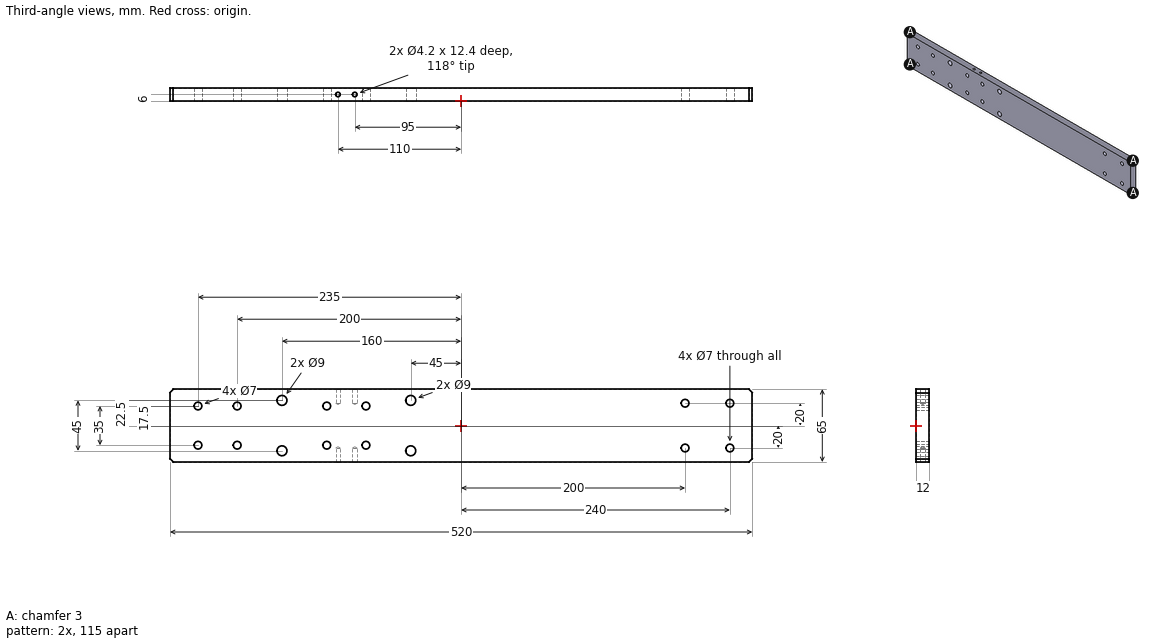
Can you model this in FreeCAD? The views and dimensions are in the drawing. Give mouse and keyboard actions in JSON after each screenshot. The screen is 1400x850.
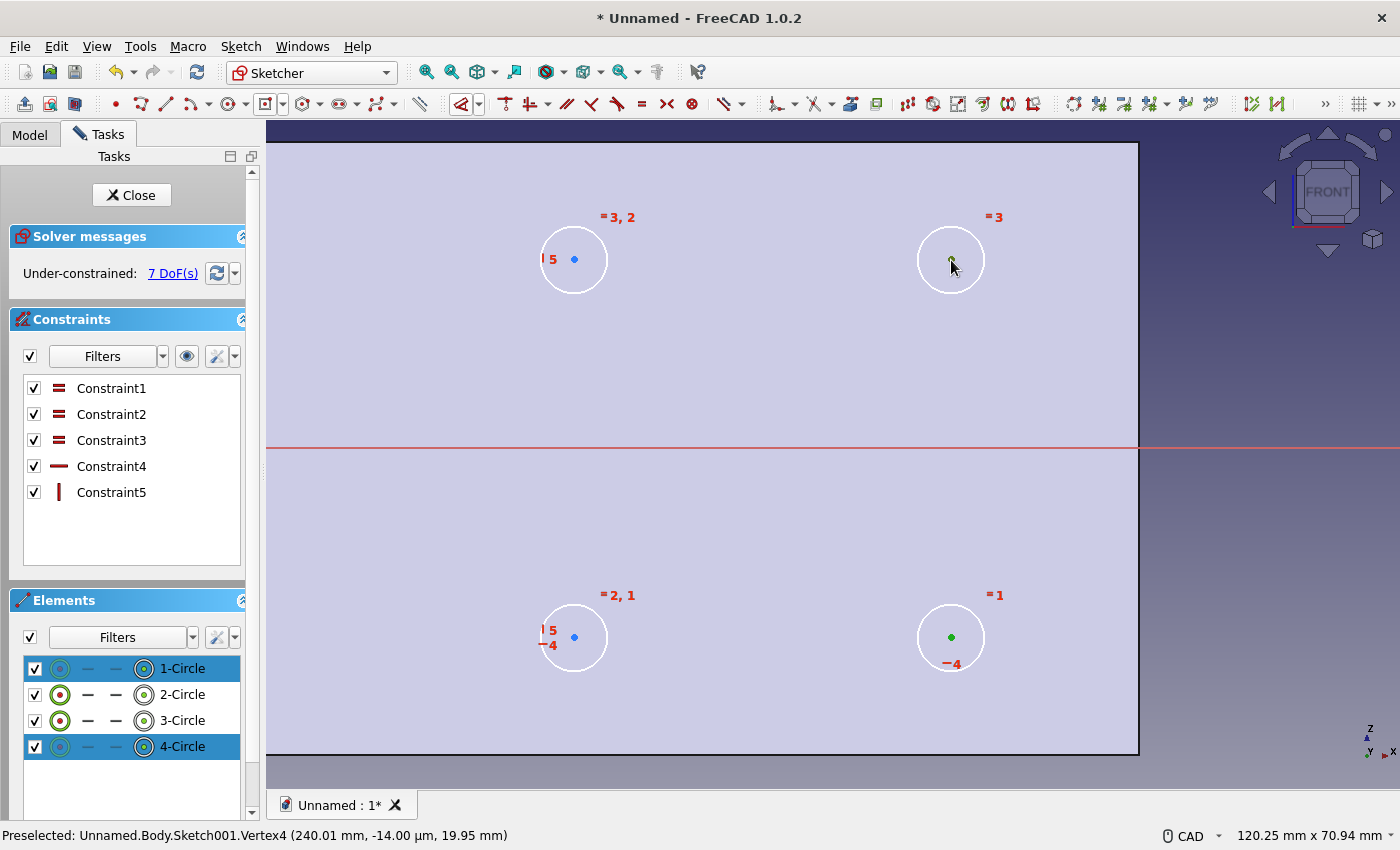
{"action": "left_click", "coordinate": [548, 104]}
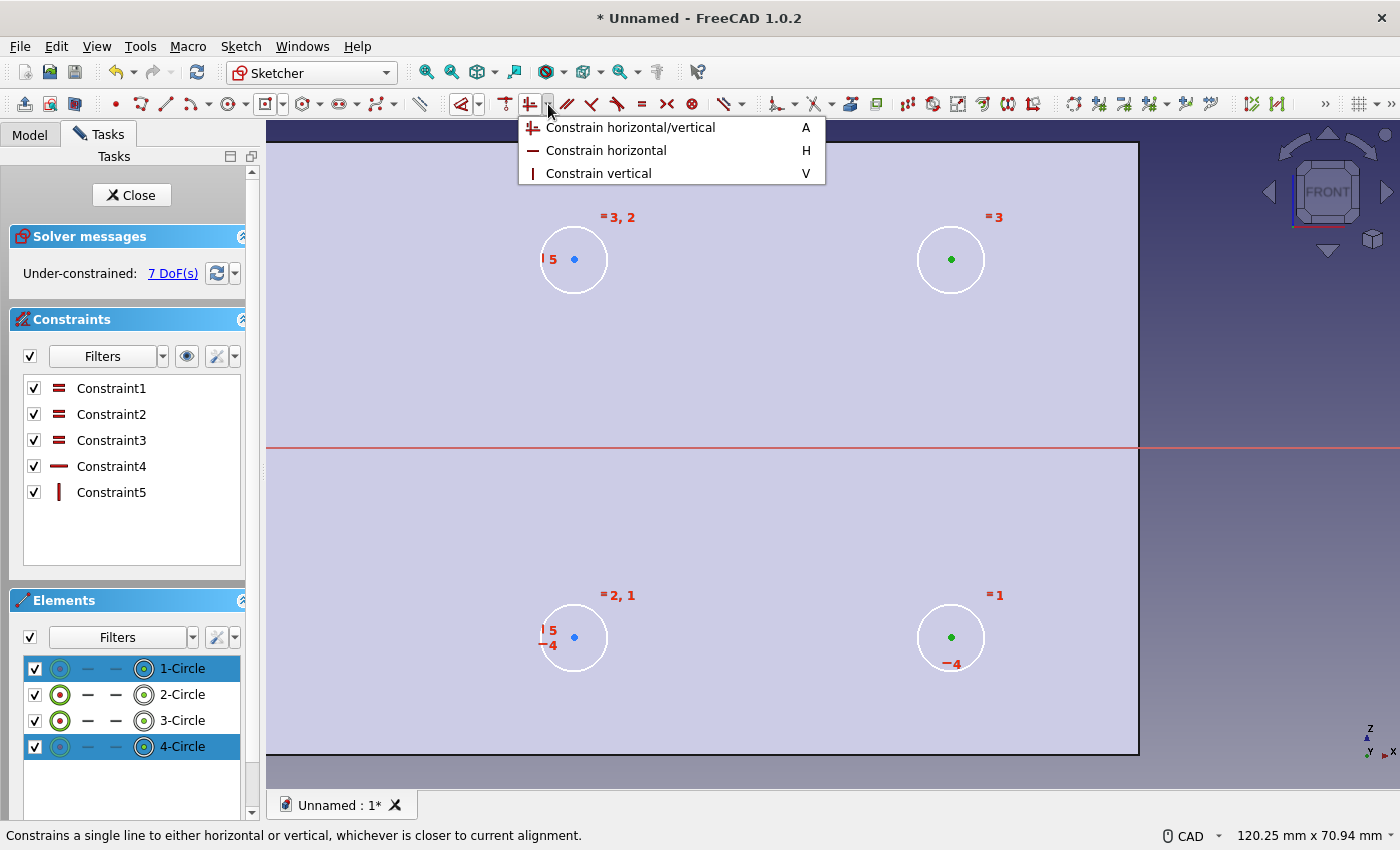
{"action": "left_click", "coordinate": [672, 174]}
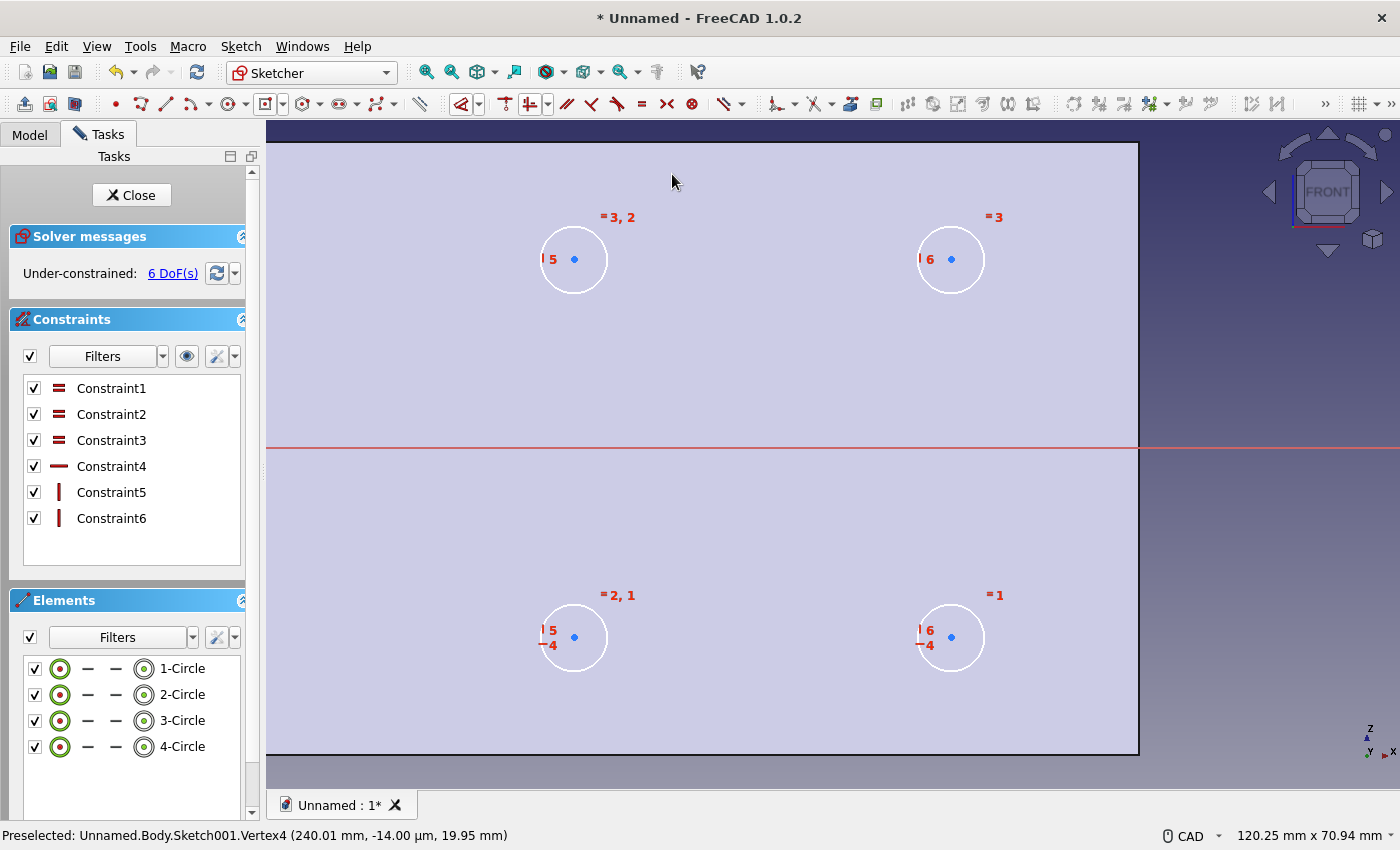
{"action": "left_click", "coordinate": [574, 260]}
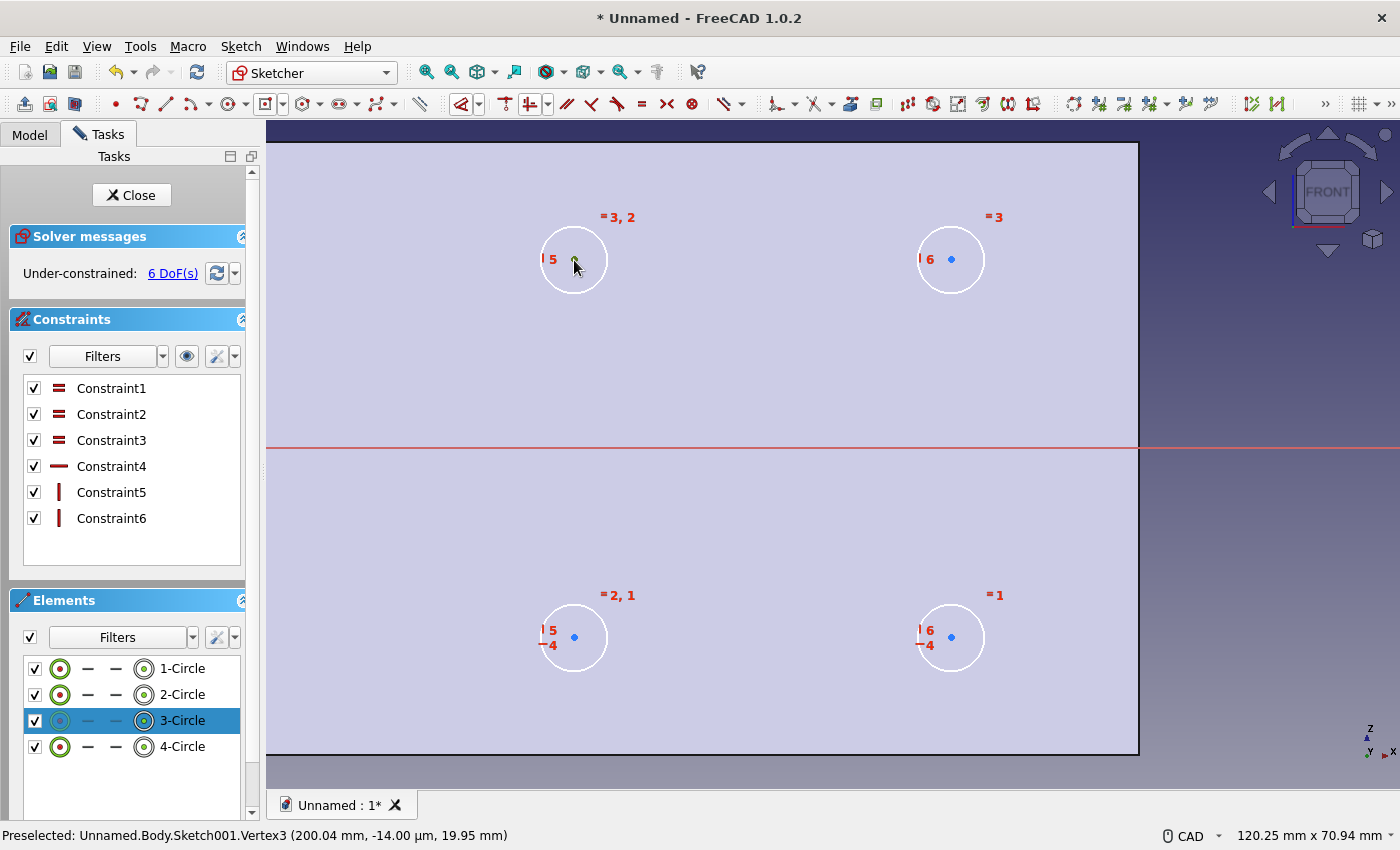
{"action": "left_click", "coordinate": [951, 260]}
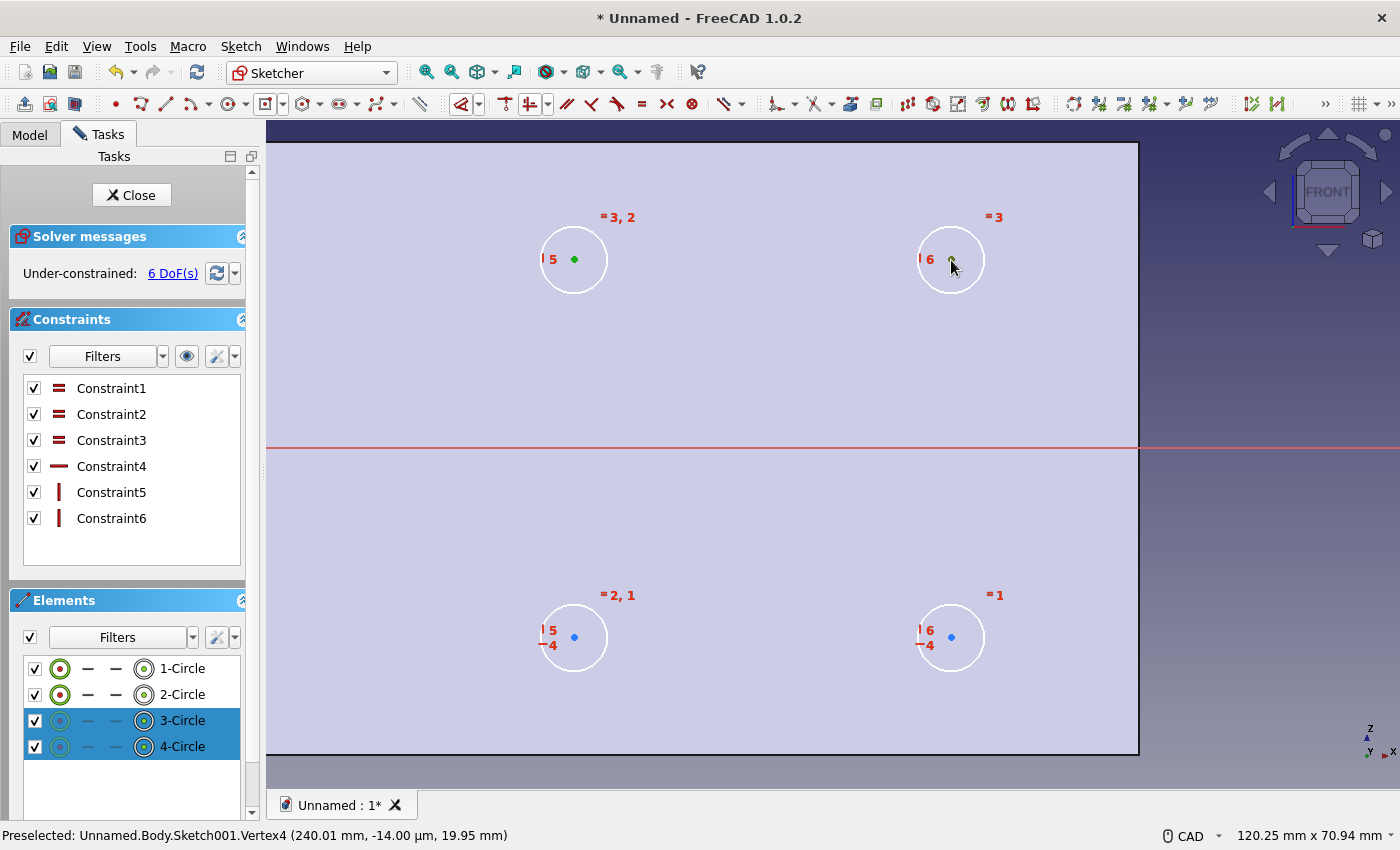
{"action": "left_click", "coordinate": [548, 104]}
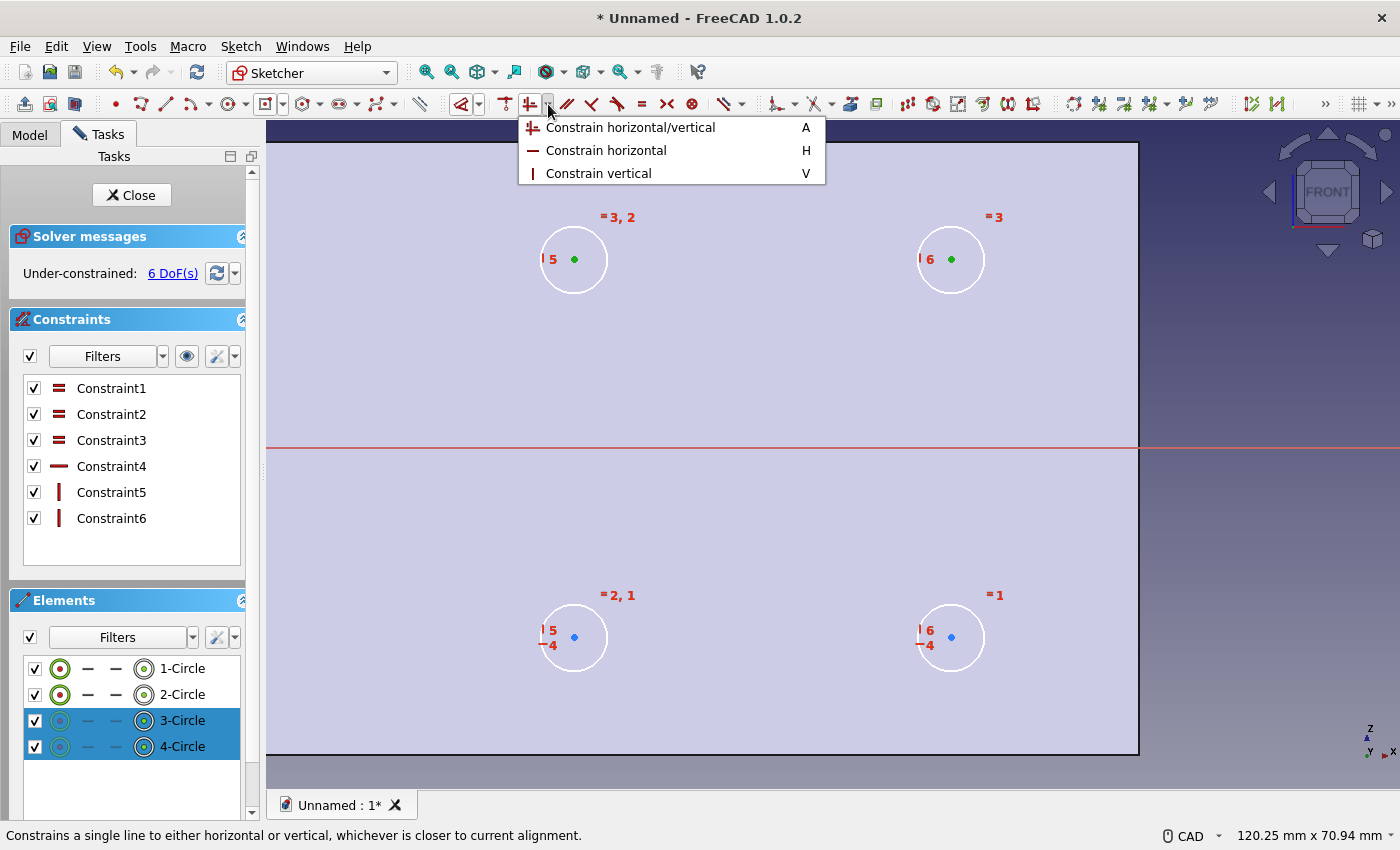
{"action": "left_click", "coordinate": [672, 150]}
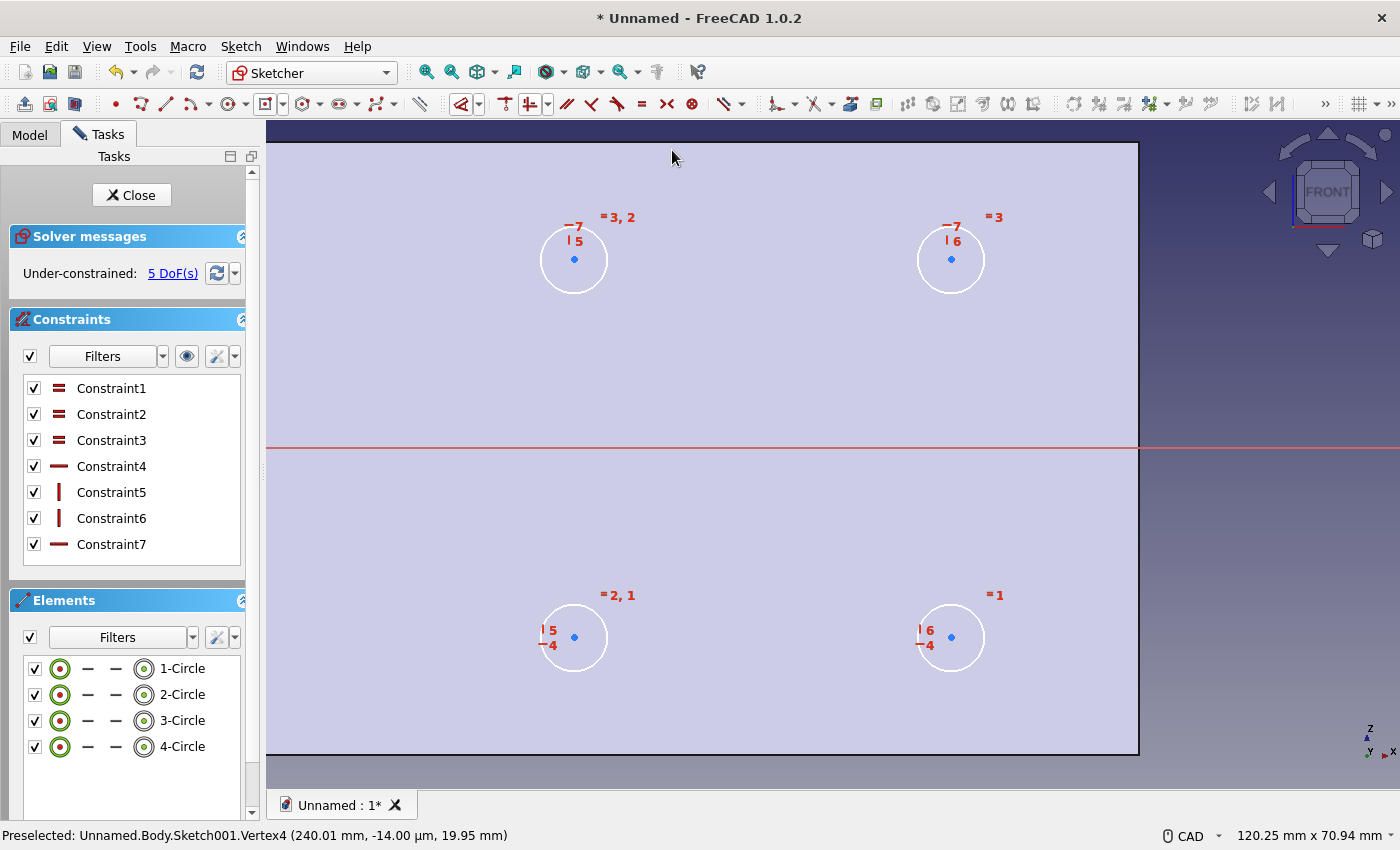
{"action": "left_click", "coordinate": [974, 614]}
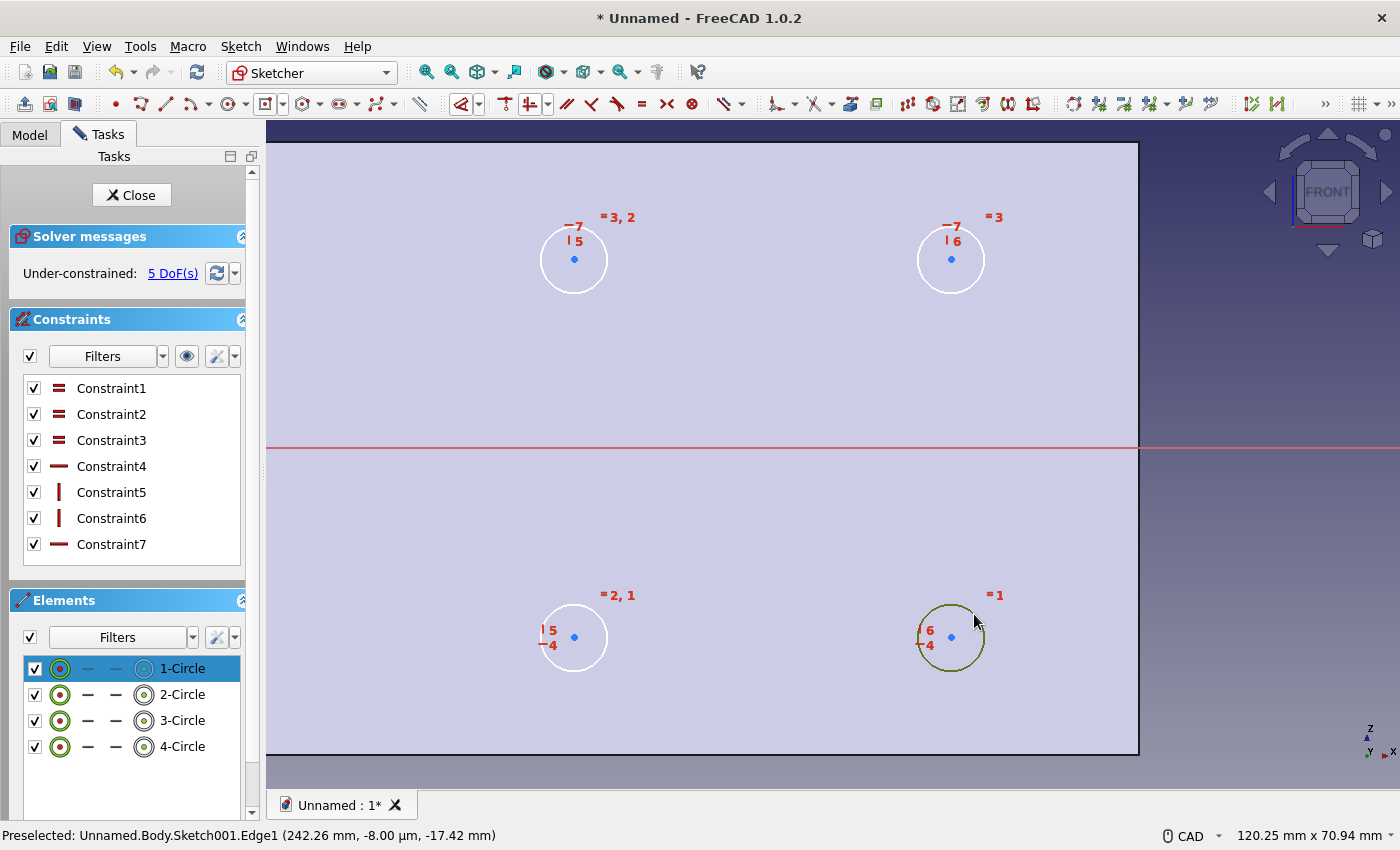
{"action": "left_click", "coordinate": [478, 104]}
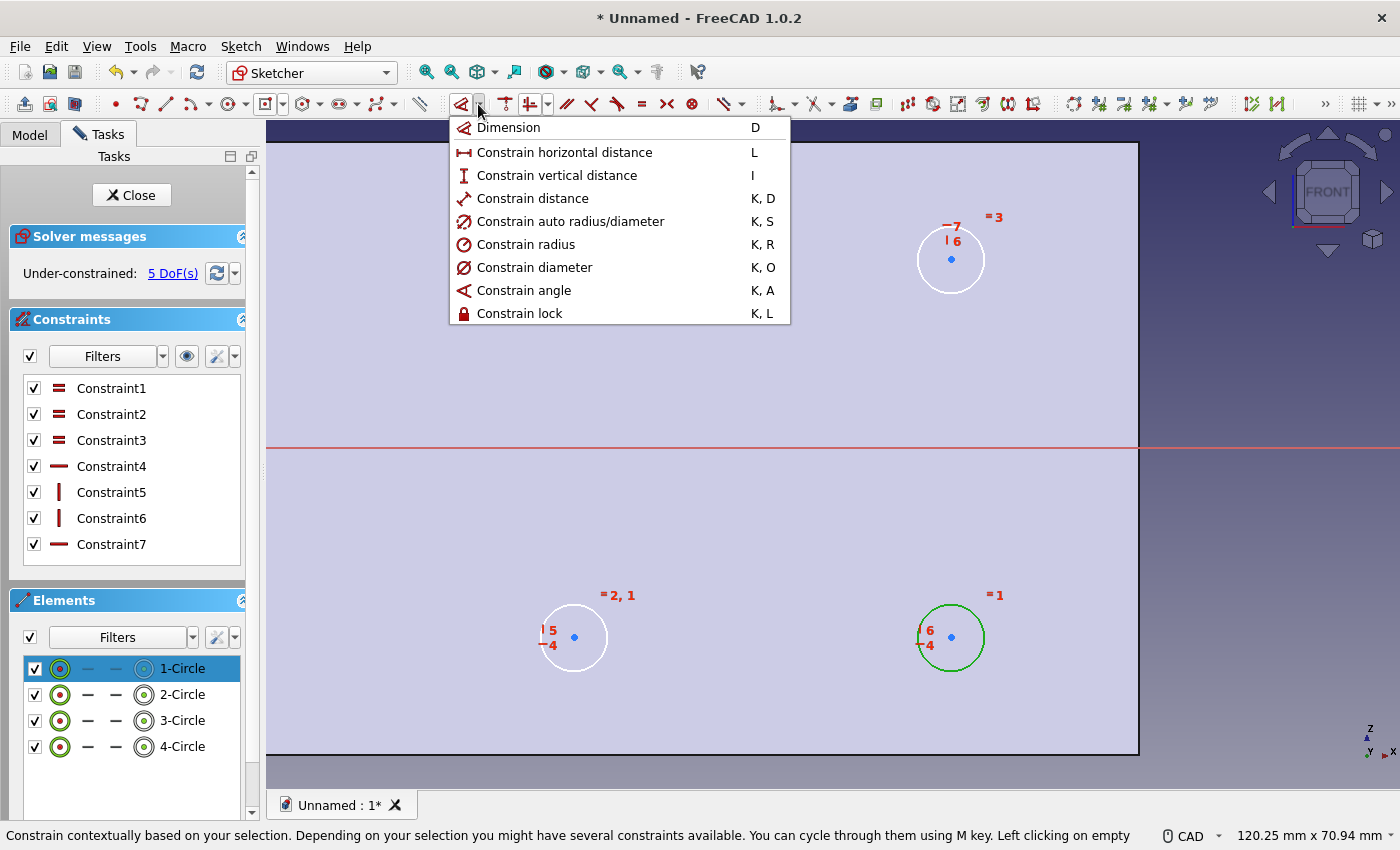
{"action": "left_click", "coordinate": [620, 268]}